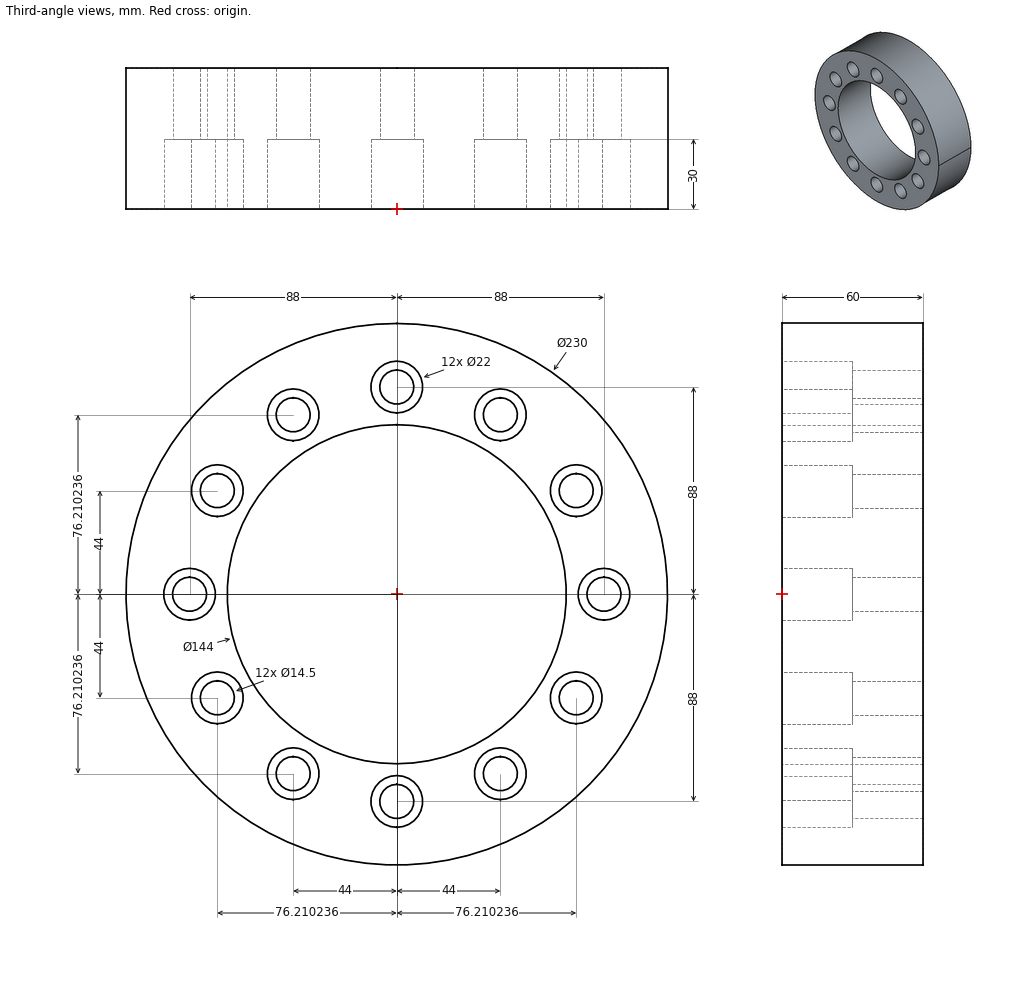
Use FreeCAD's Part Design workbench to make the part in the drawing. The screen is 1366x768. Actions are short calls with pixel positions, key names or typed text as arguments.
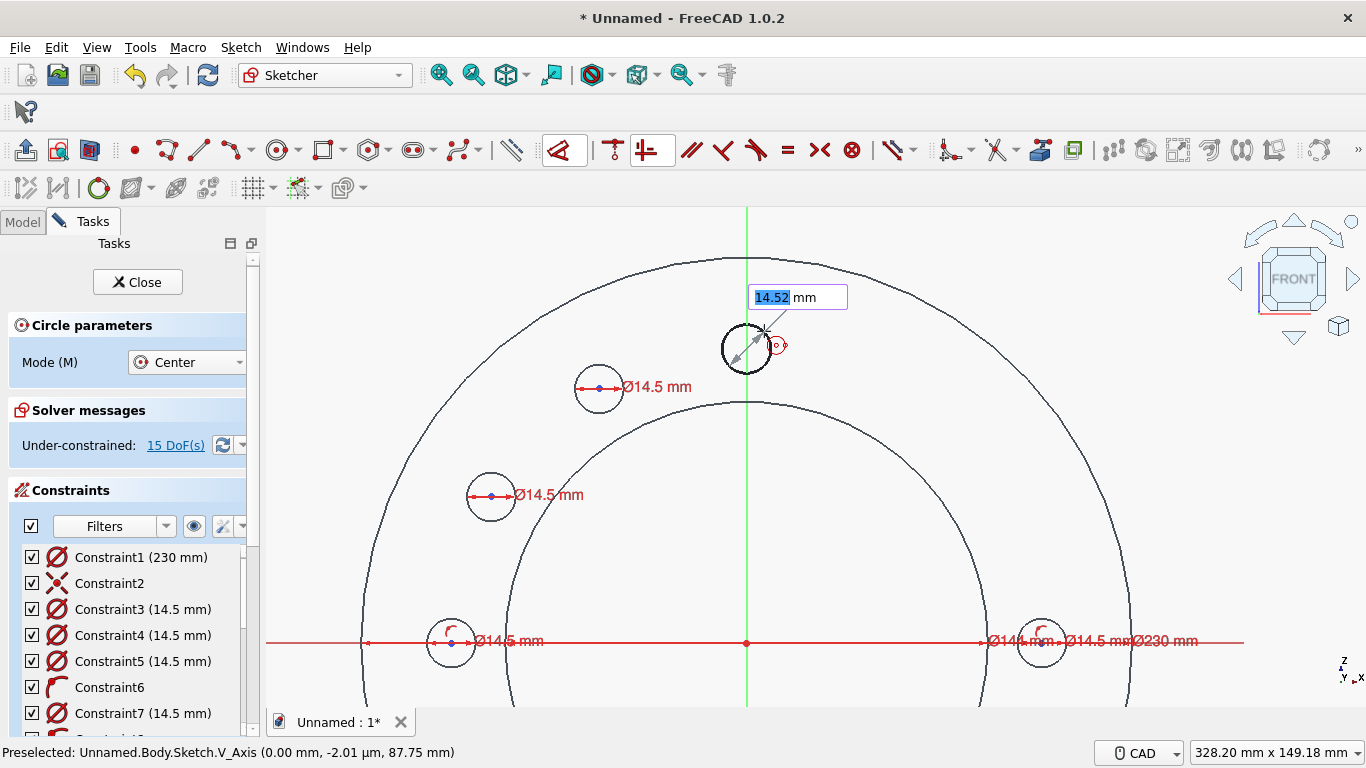
text(14.5)
key(Return)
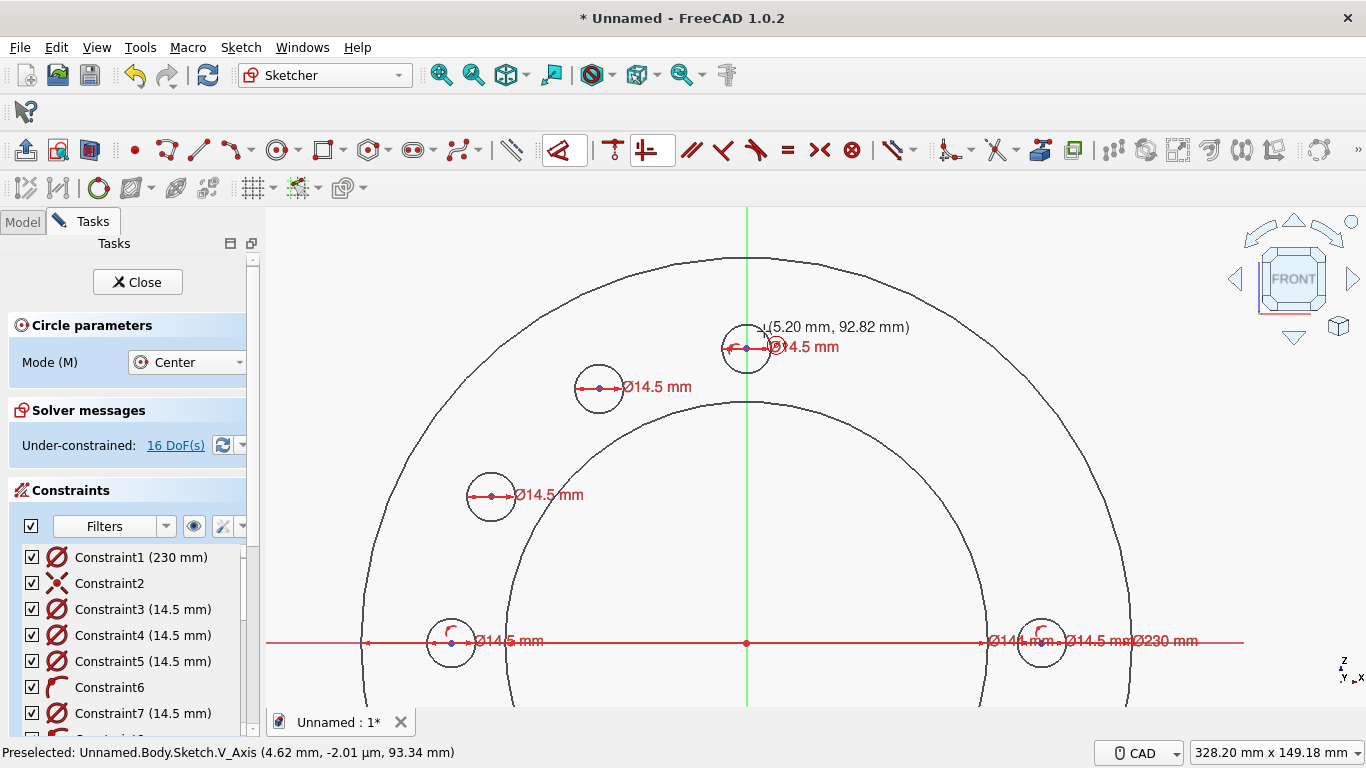
click(894, 388)
move(911, 371)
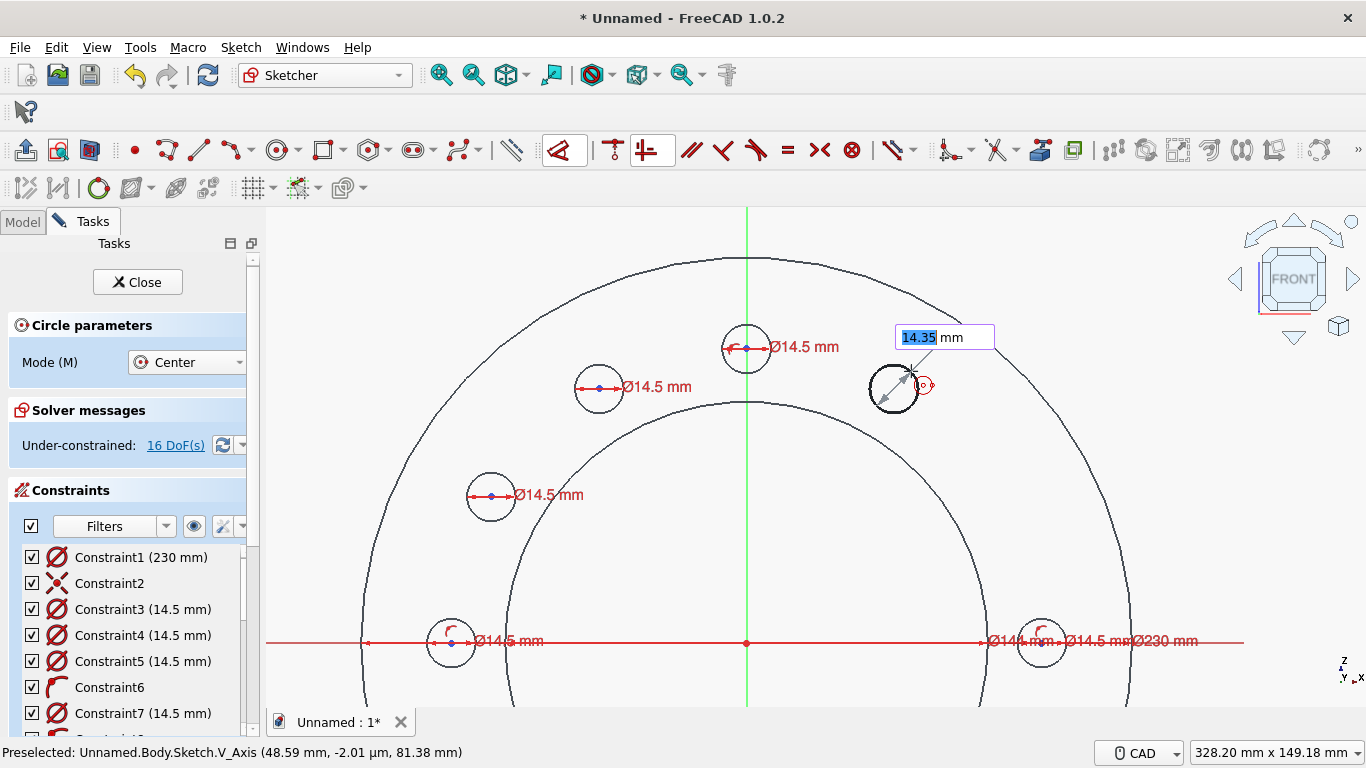
text(14.5)
key(Return)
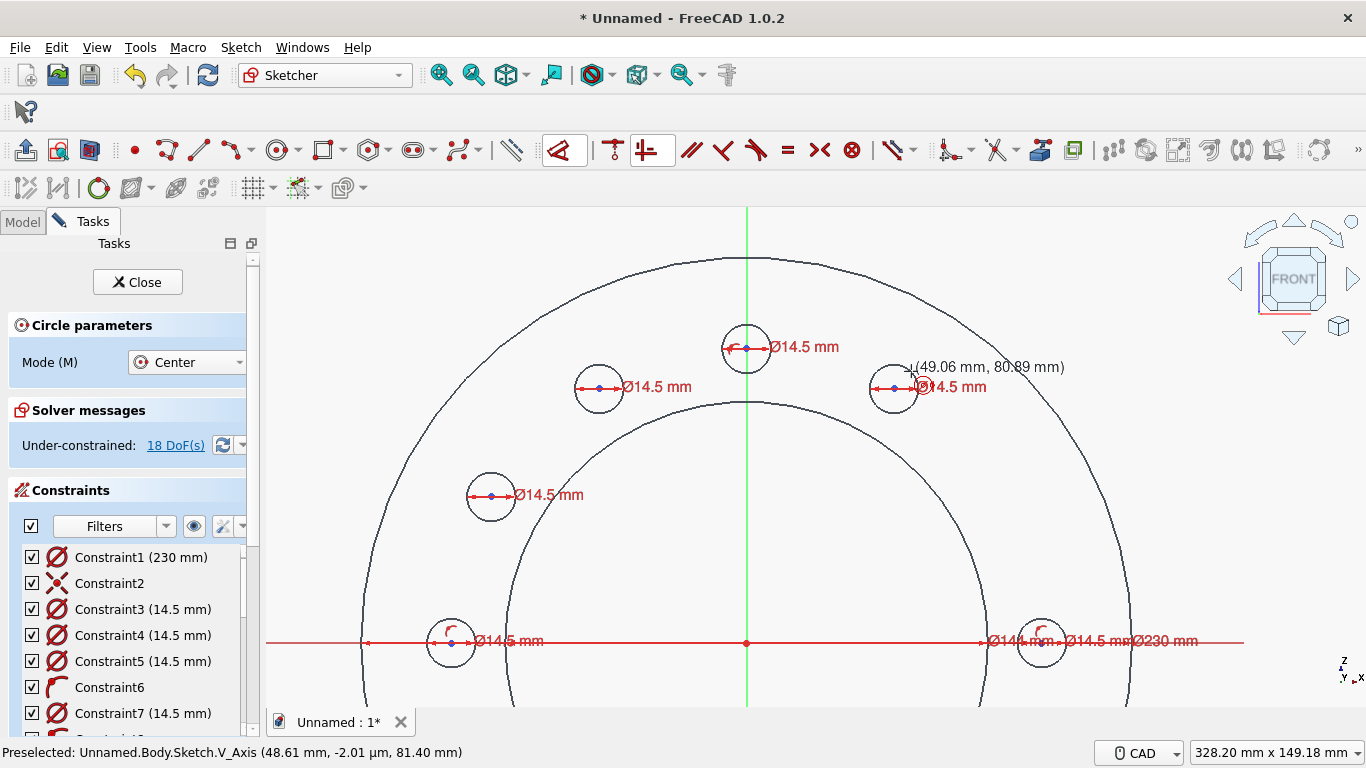
click(1002, 496)
move(1019, 478)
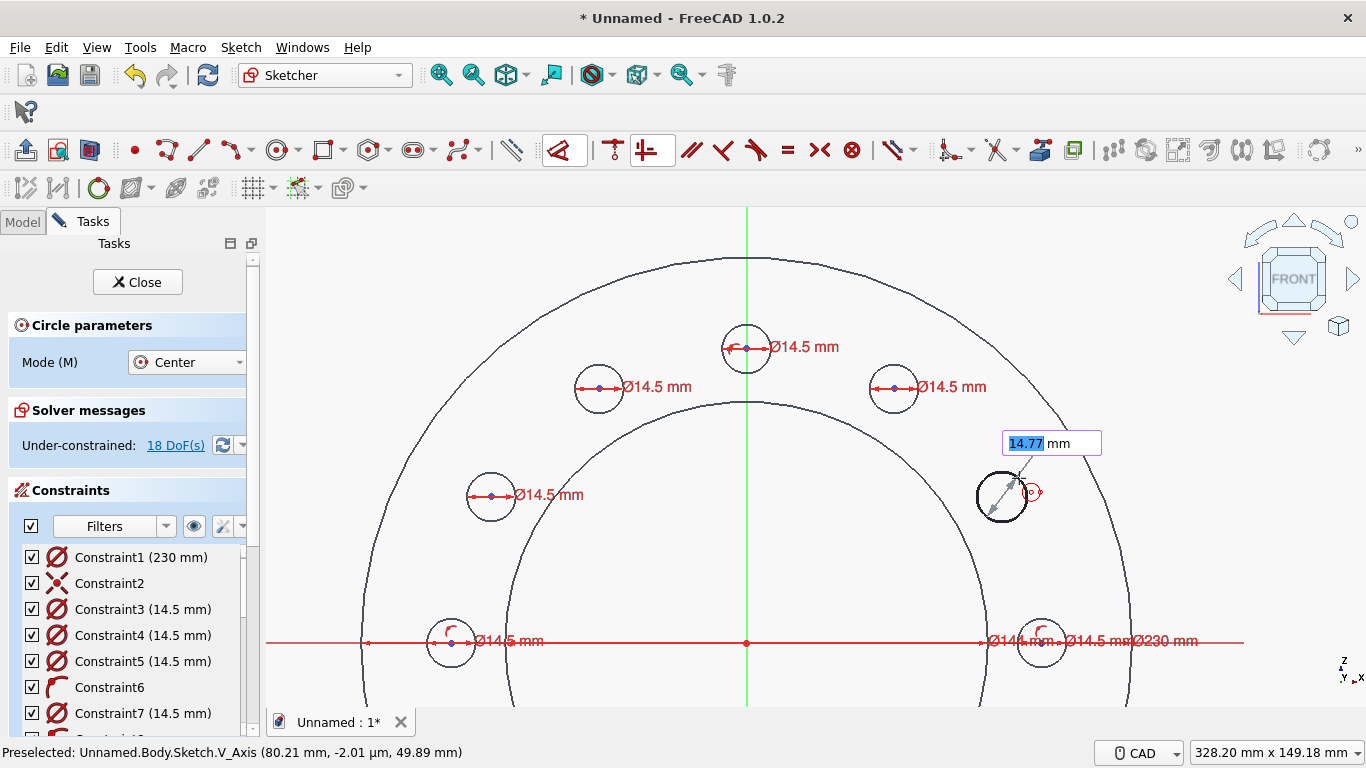
text(14.5)
key(Return)
key(Escape)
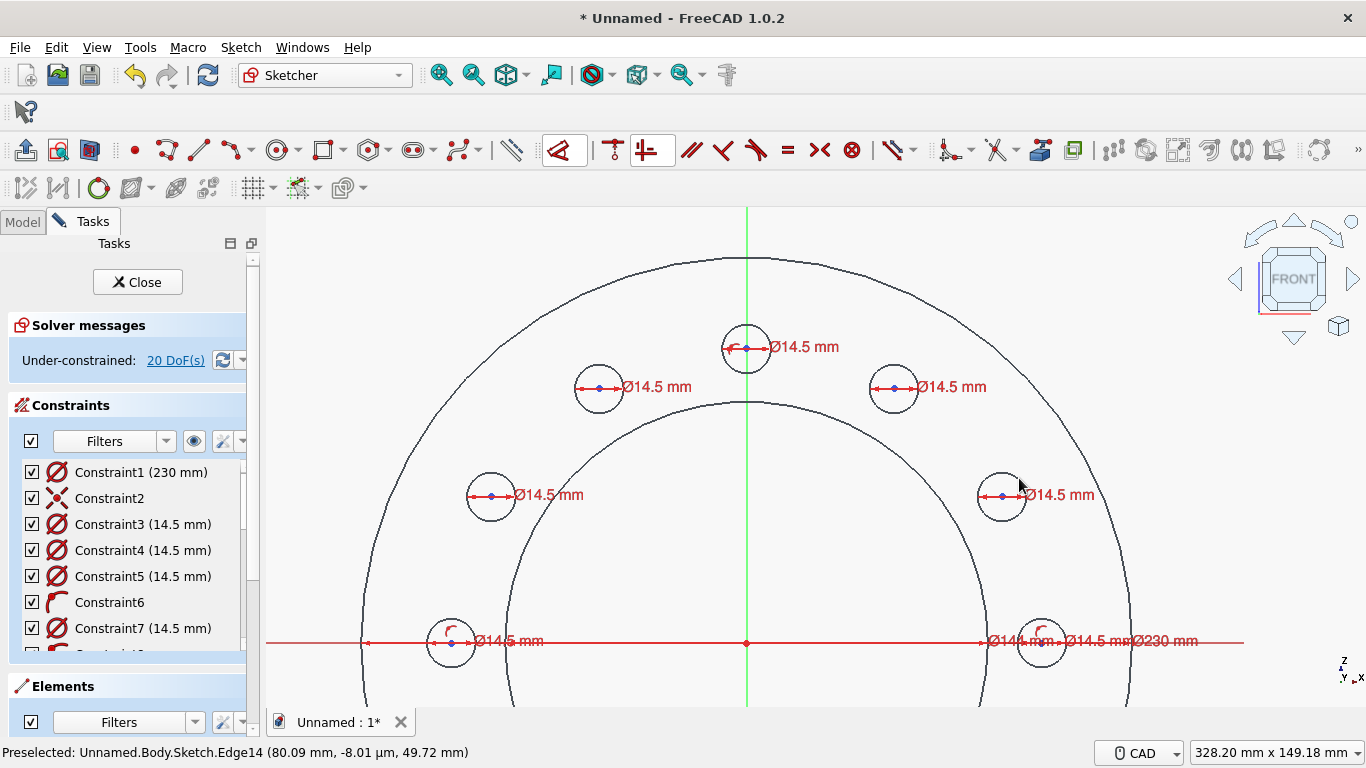
scroll(748, 349, down, 5)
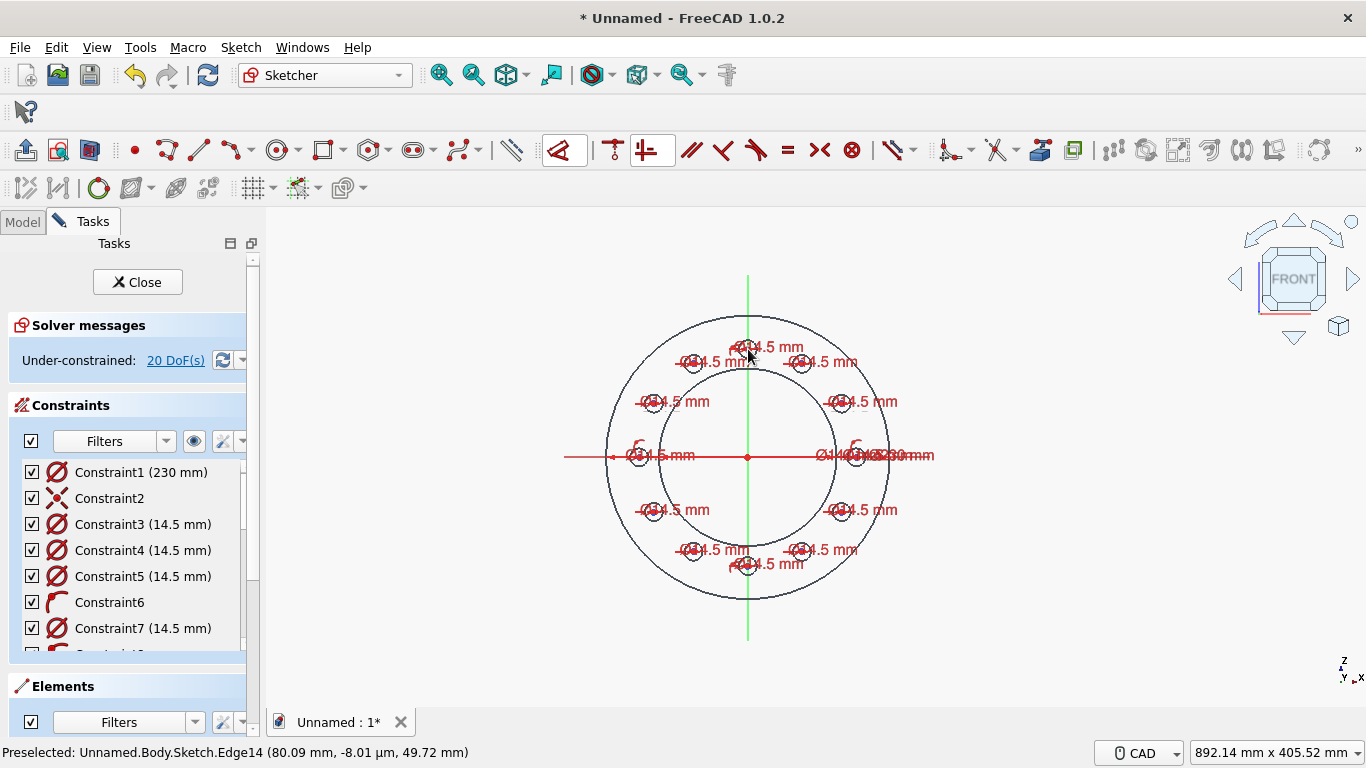
click(654, 512)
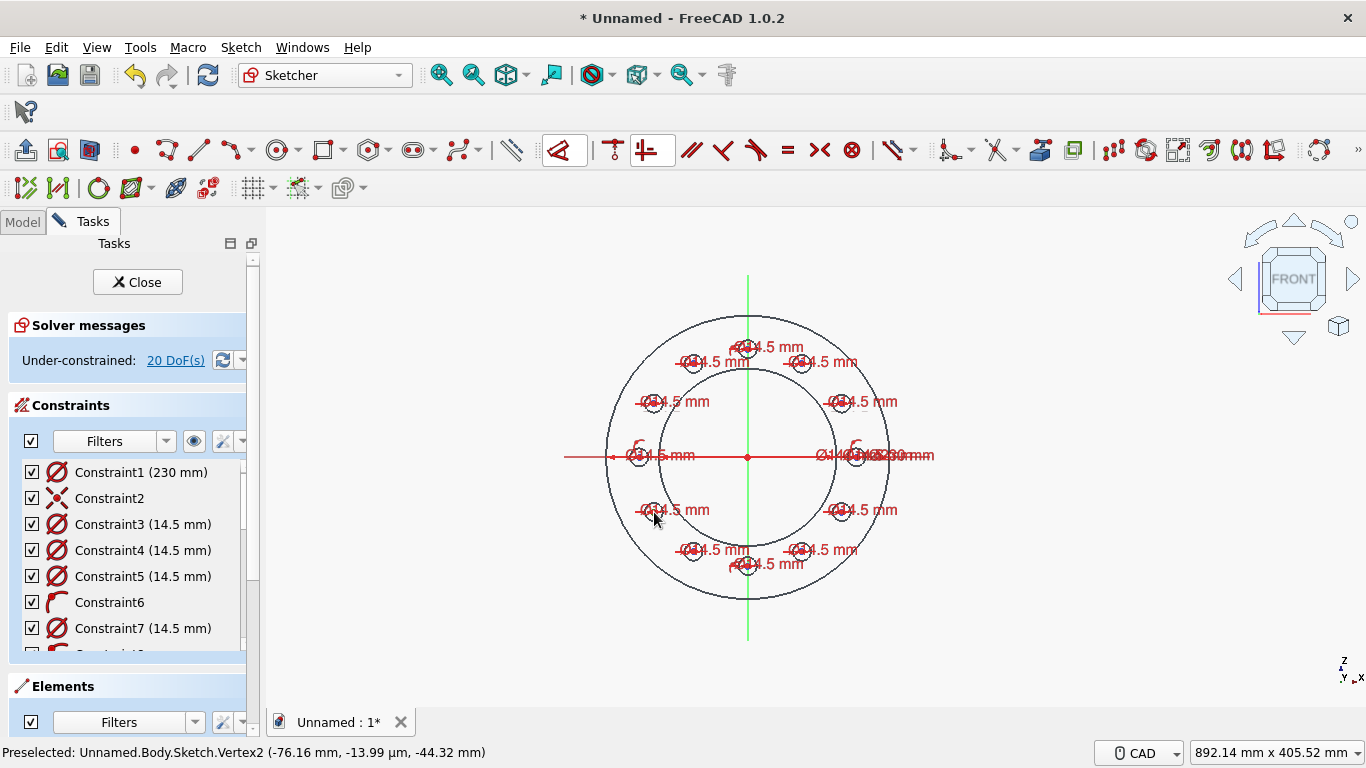
click(654, 404)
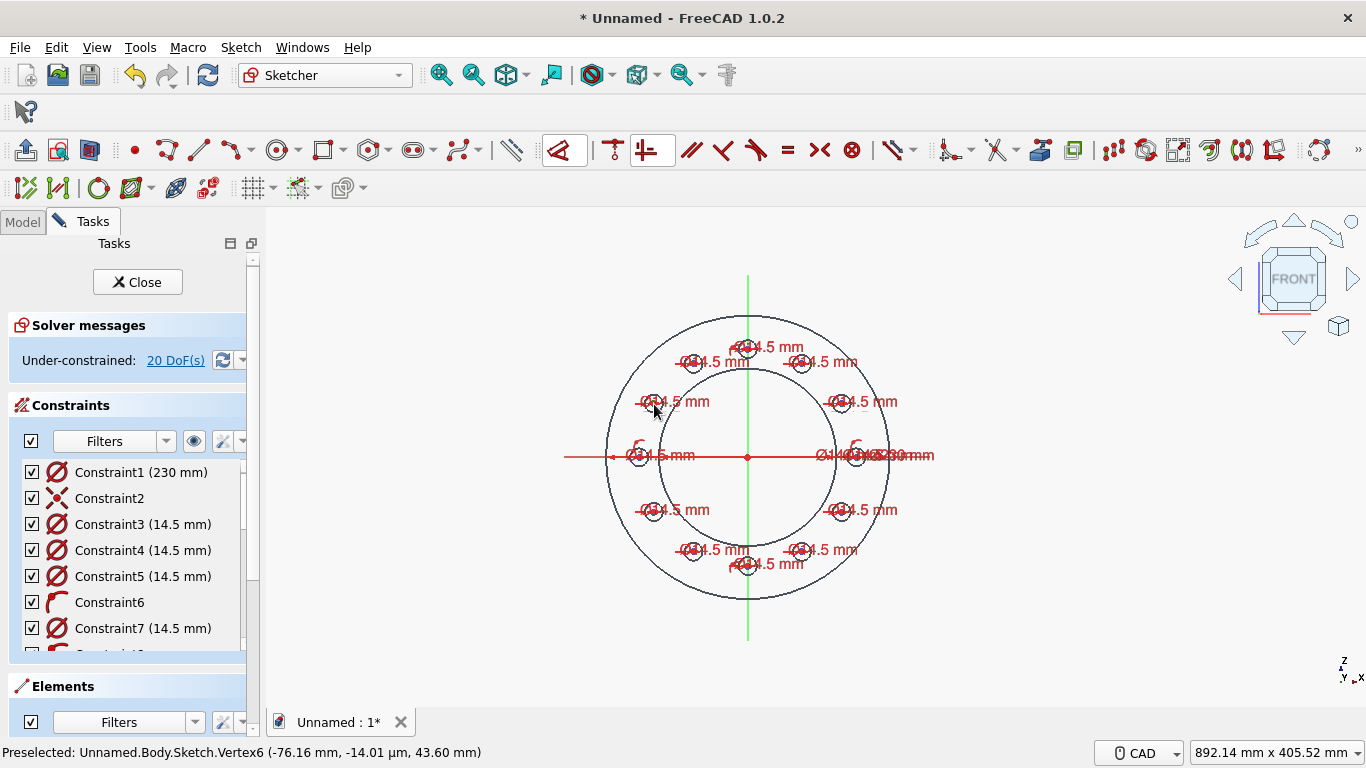
key(v)